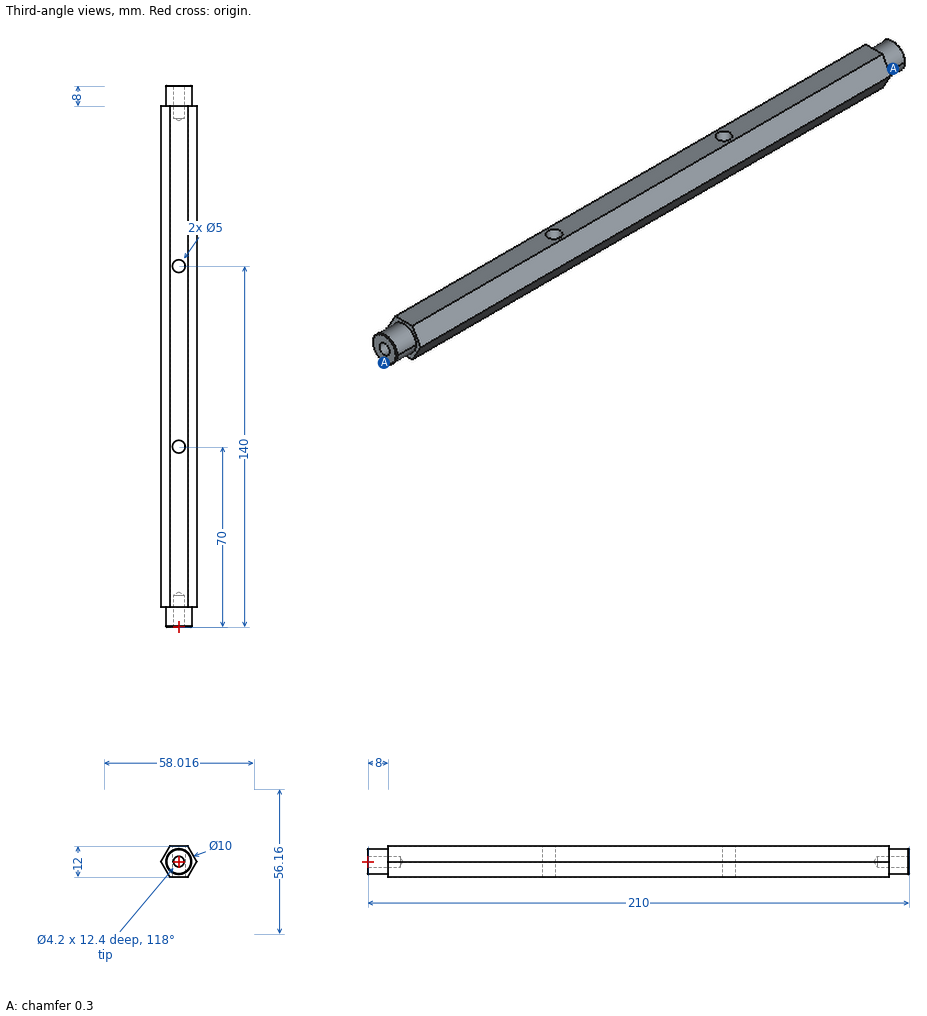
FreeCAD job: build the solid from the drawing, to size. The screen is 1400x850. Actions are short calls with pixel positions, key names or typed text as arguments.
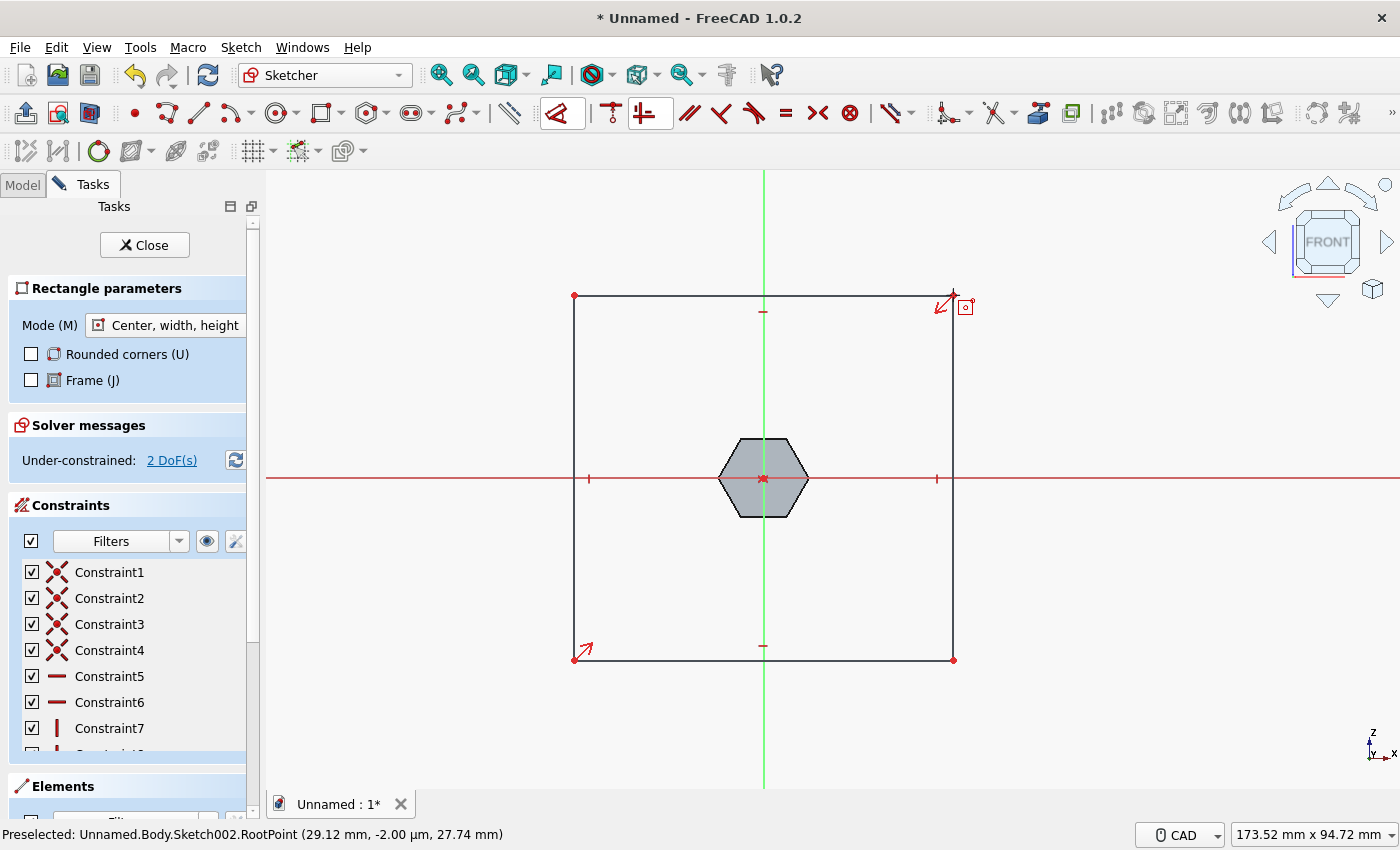
key(g)
key(c)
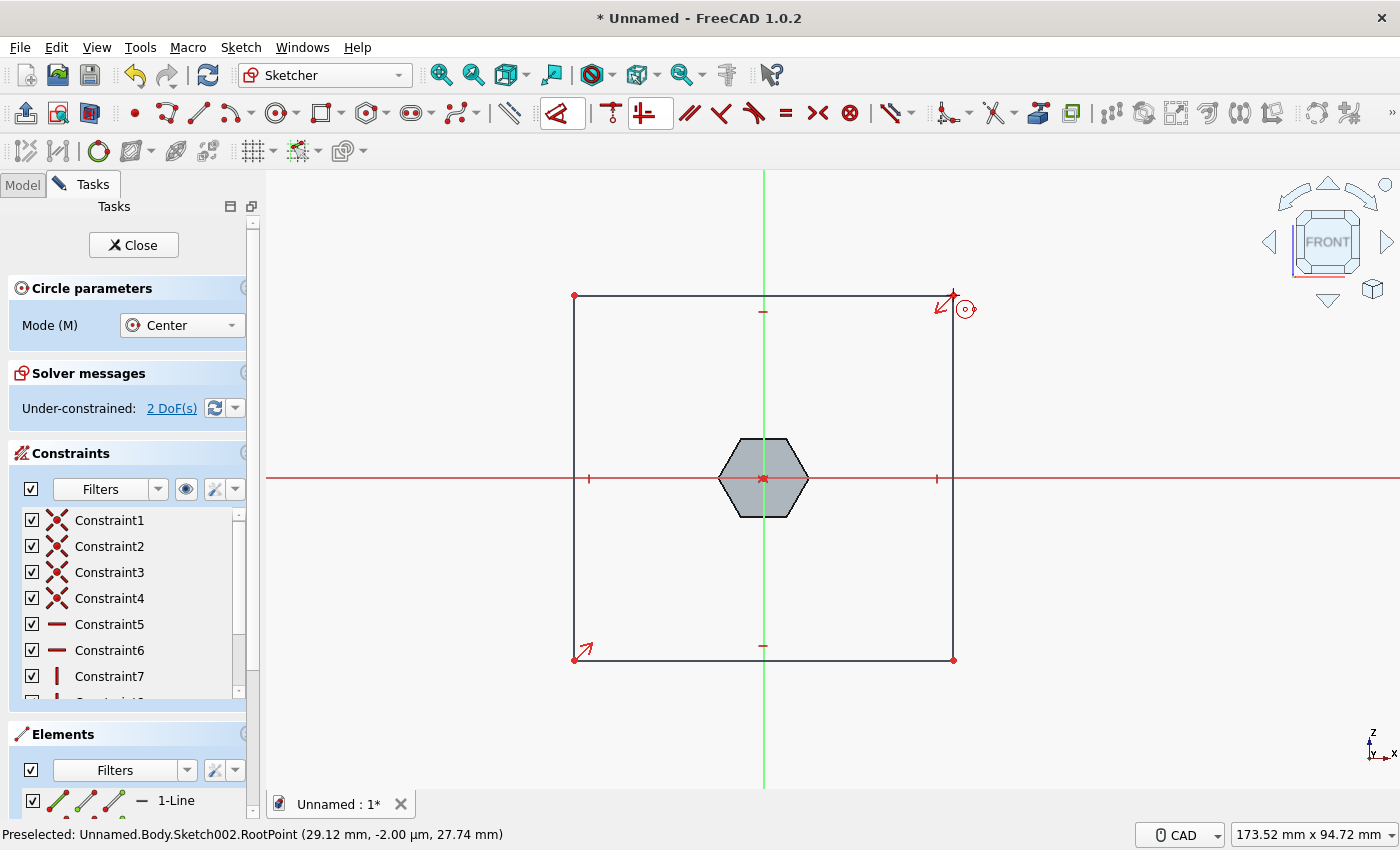
click(764, 478)
click(787, 455)
key(Escape)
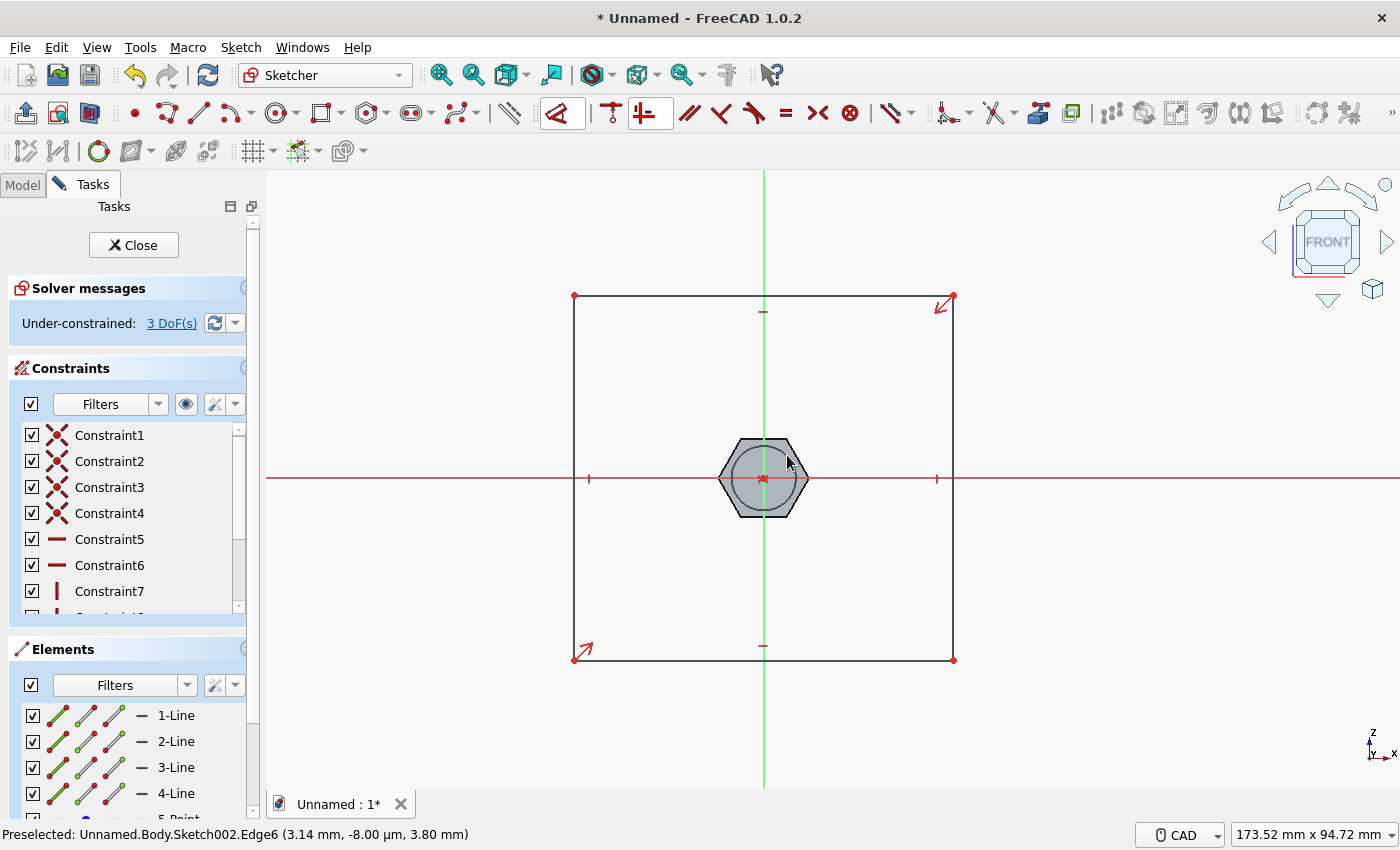
click(786, 455)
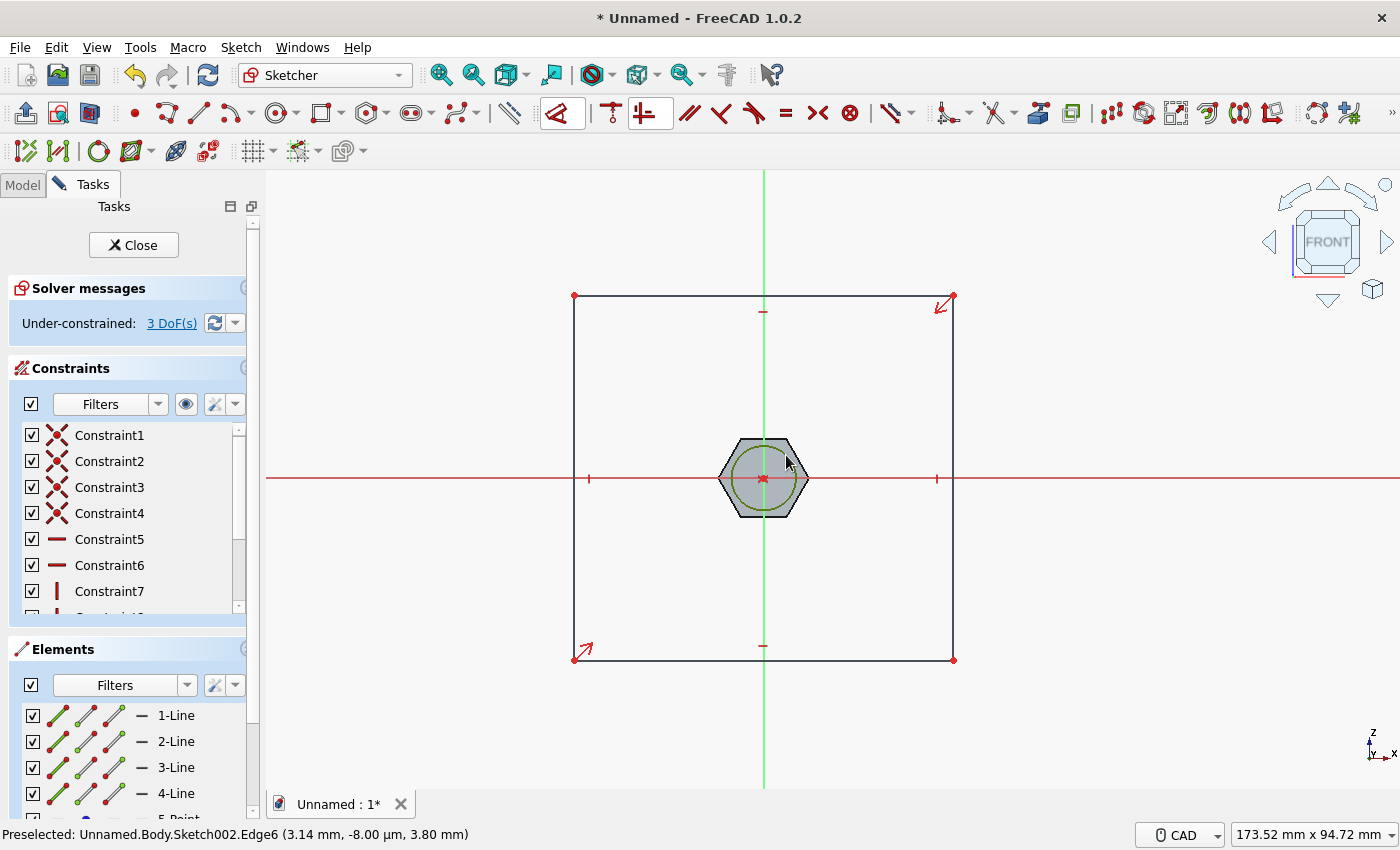
key(k)
key(o)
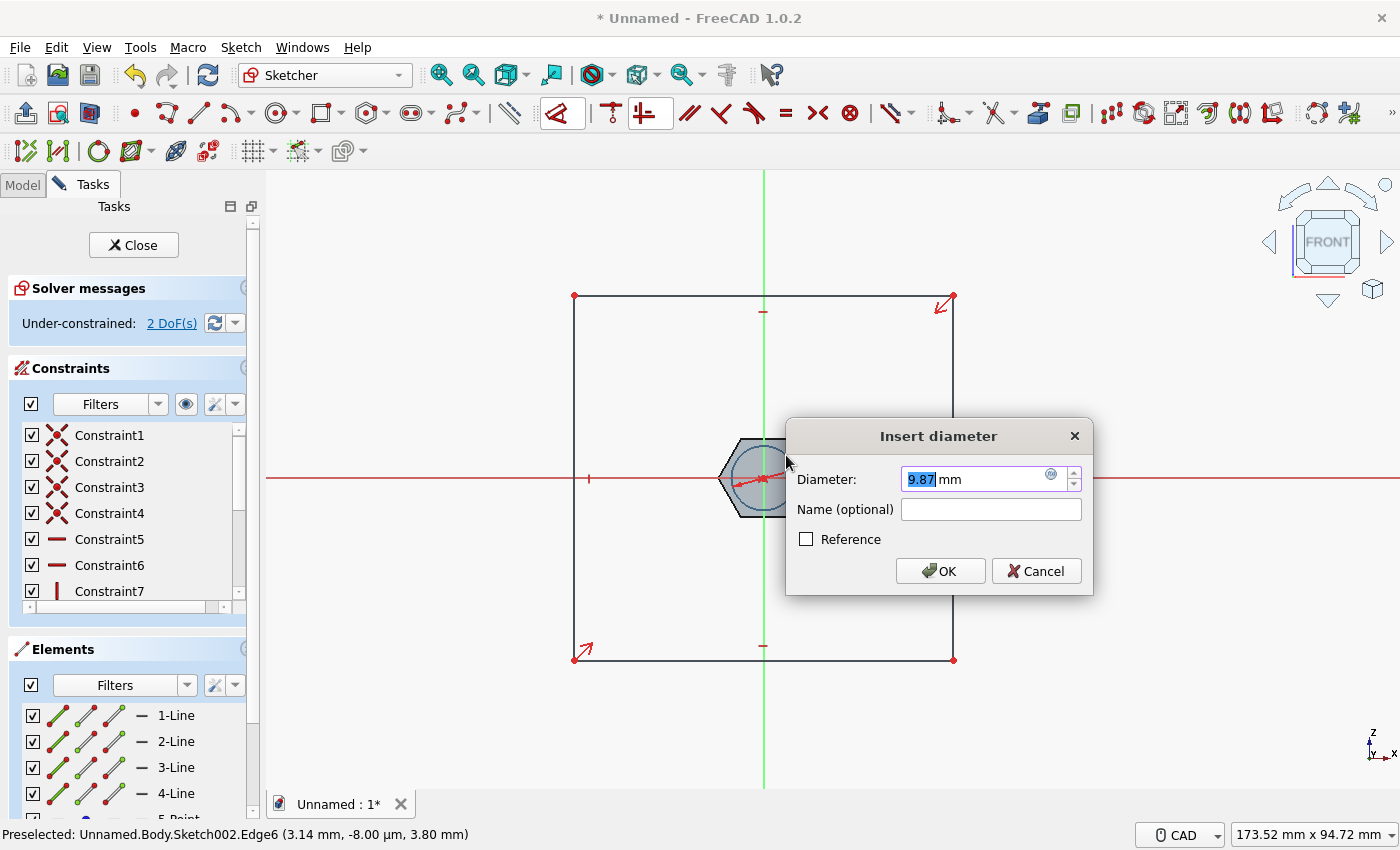
text(10)
key(Return)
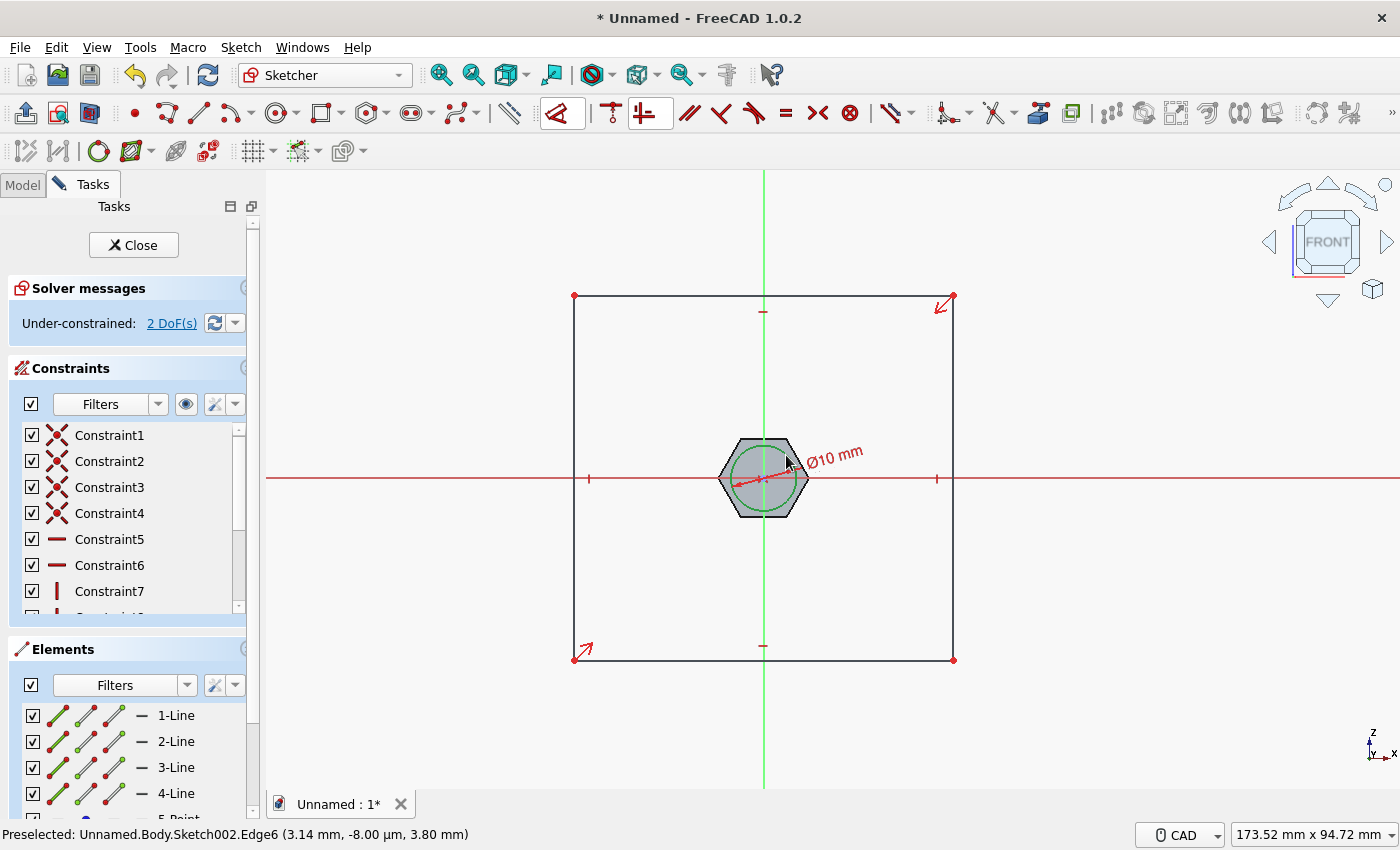
click(953, 551)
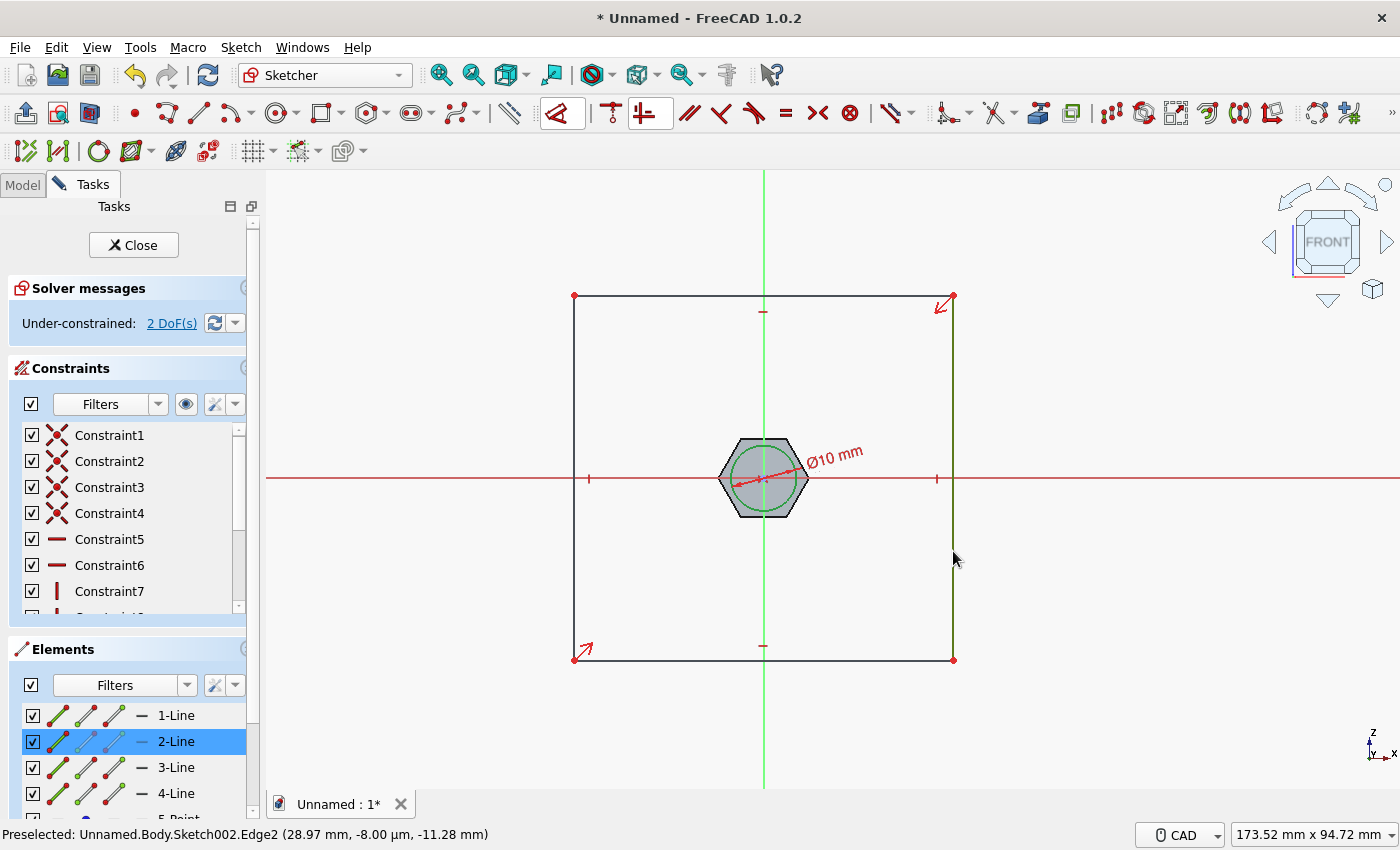
key(i)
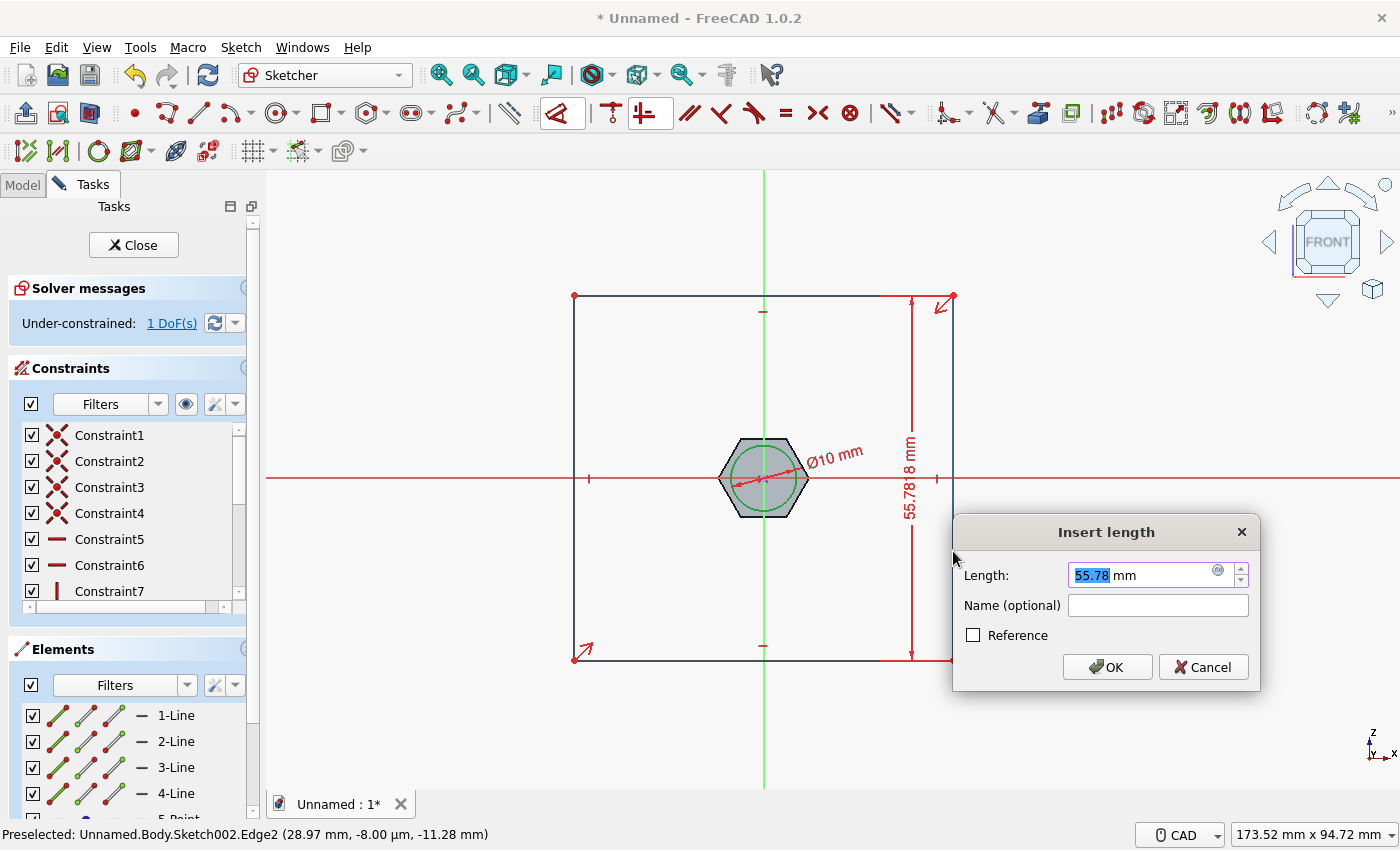
text(56.16)
key(Return)